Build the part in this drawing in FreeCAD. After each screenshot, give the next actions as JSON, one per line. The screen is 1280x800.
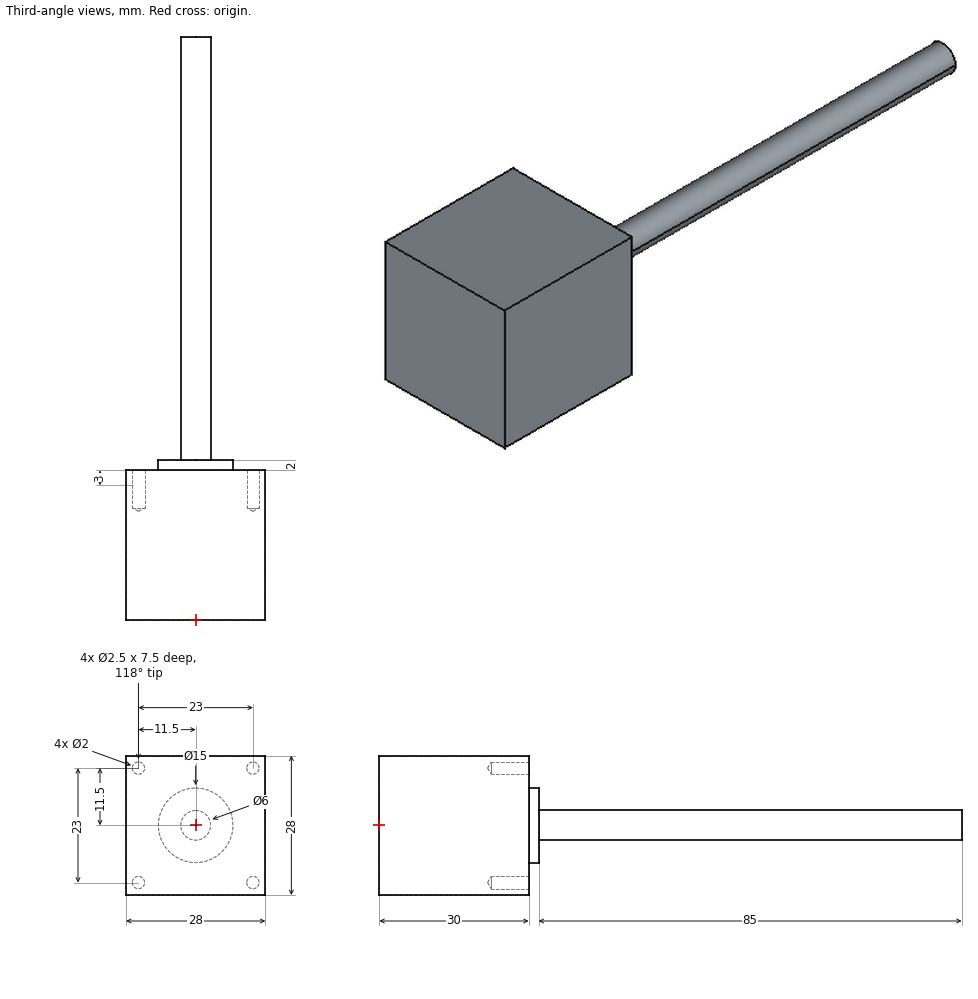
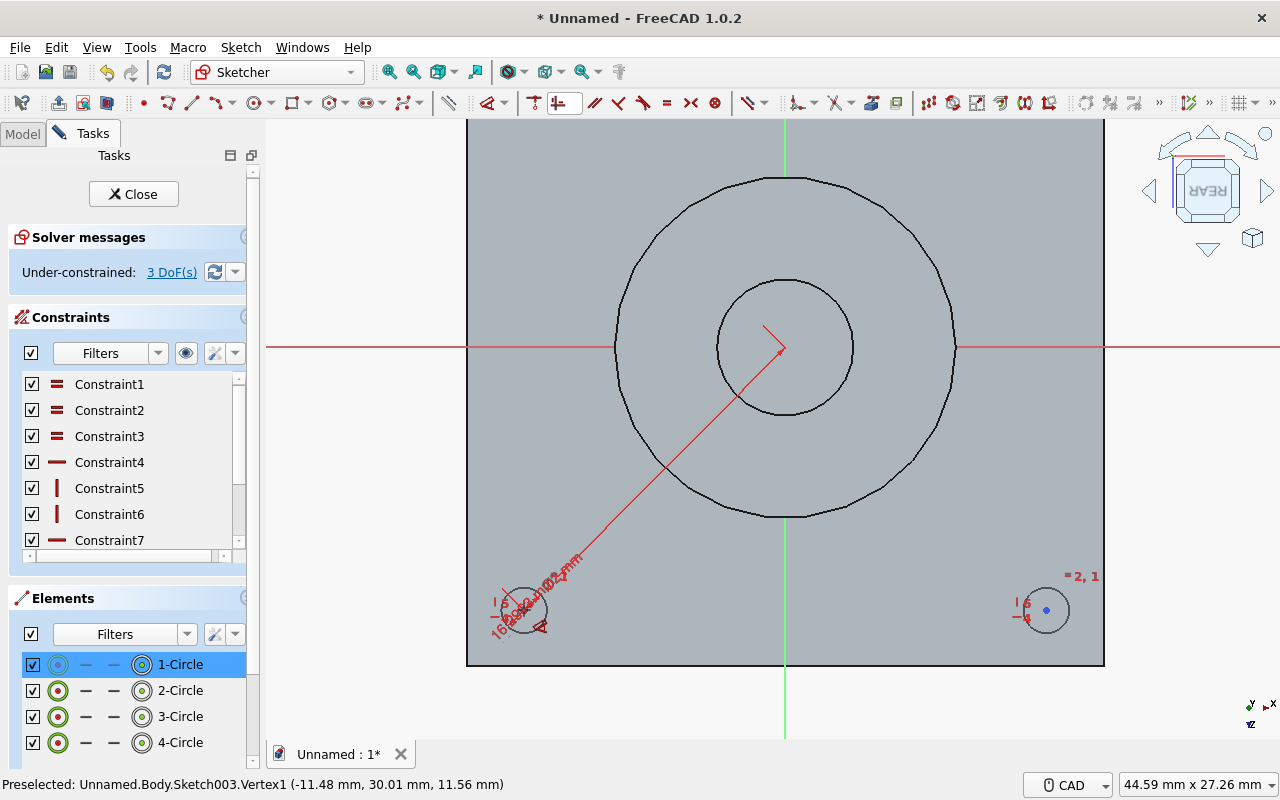
{"action": "left_click", "coordinate": [1046, 610]}
{"action": "left_click", "coordinate": [665, 644]}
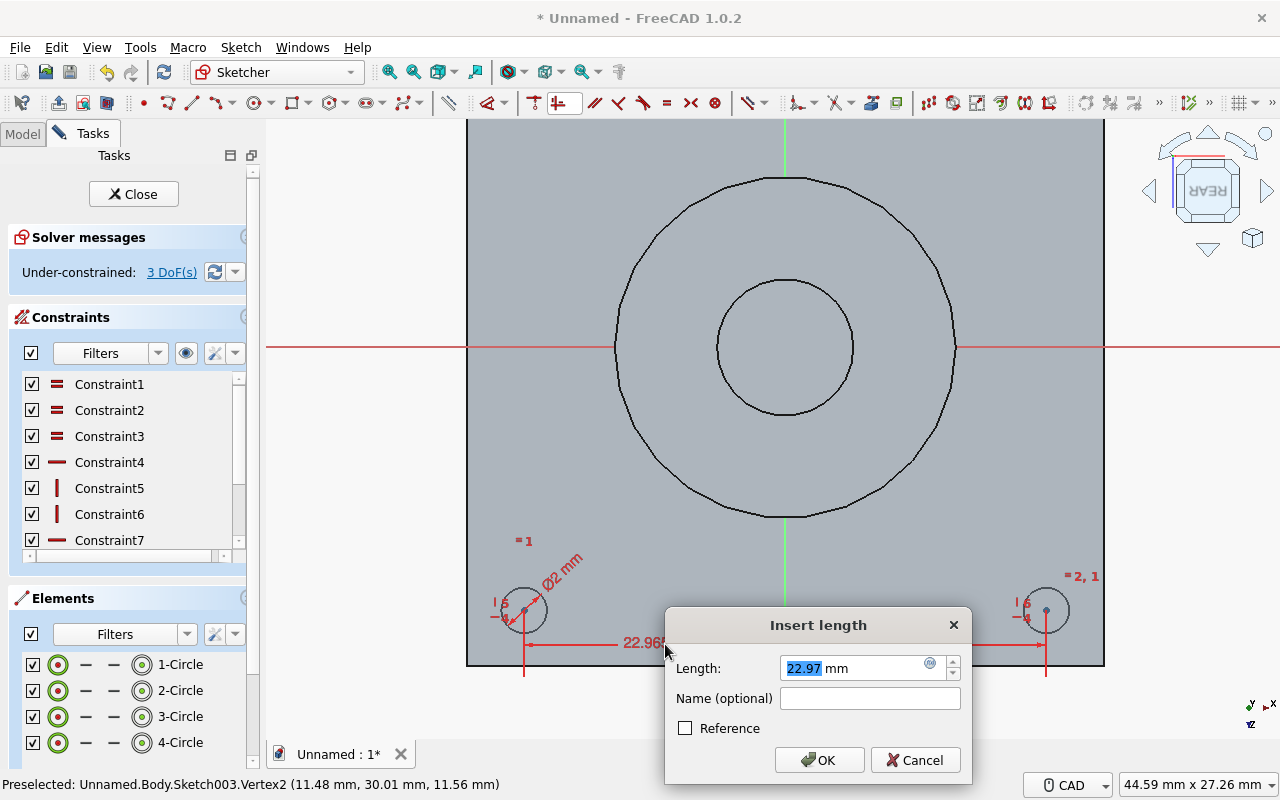
{"action": "type", "text": "23"}
{"action": "key", "text": "Return"}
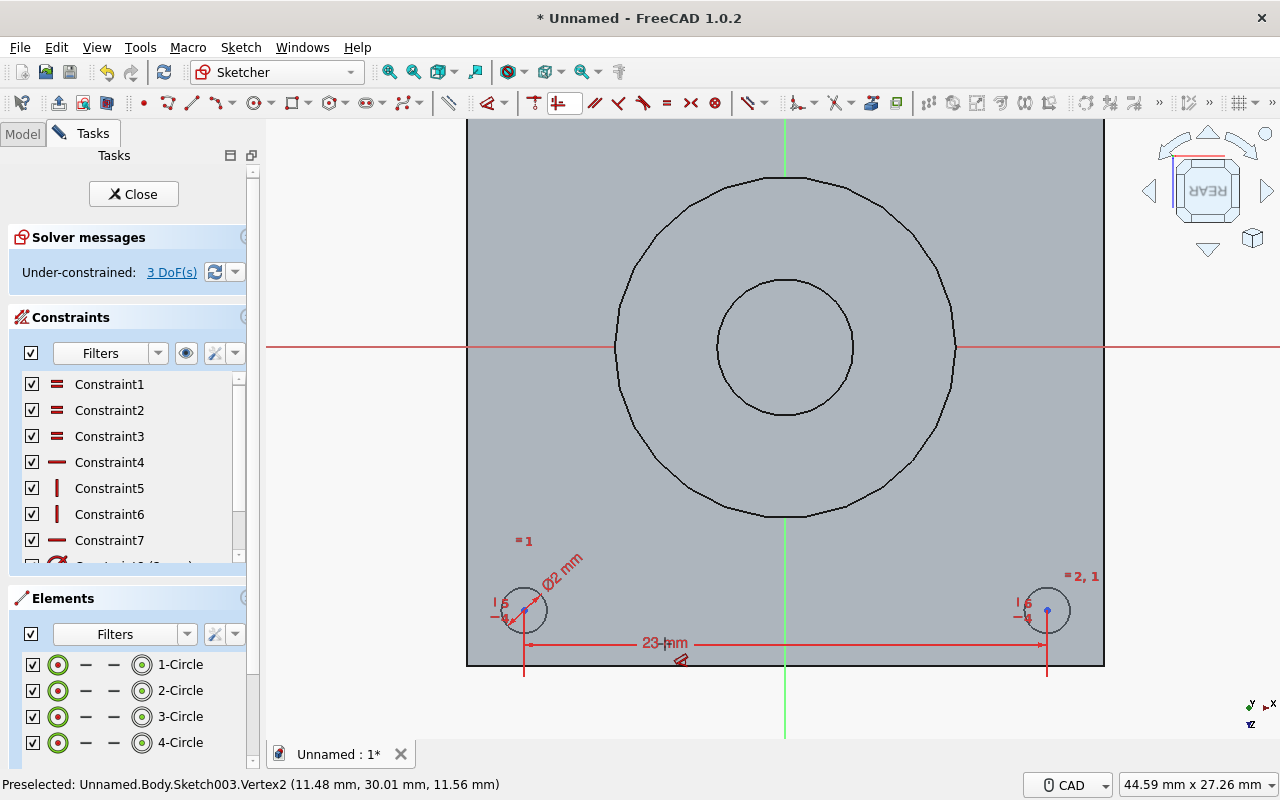
{"action": "left_click", "coordinate": [524, 610]}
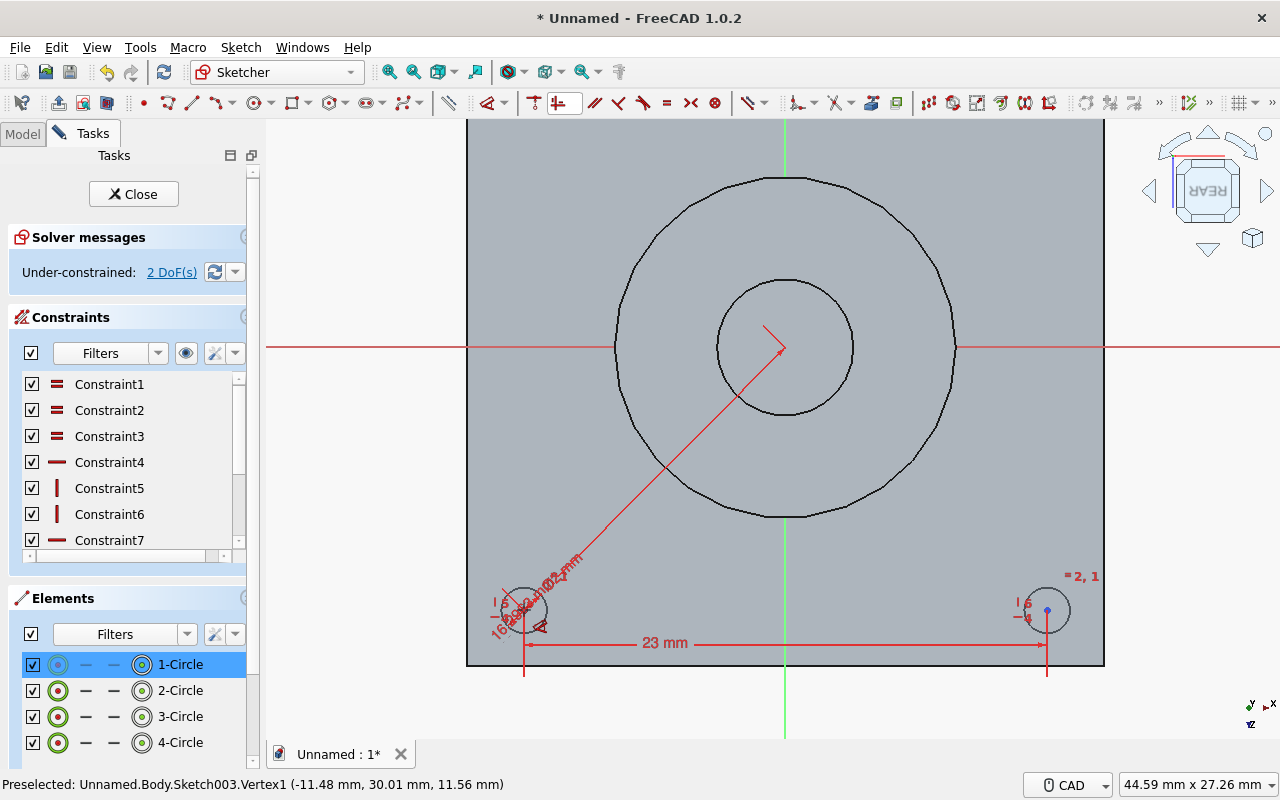
{"action": "scroll", "coordinate": [540, 595], "scroll_direction": "down", "scroll_amount": 2}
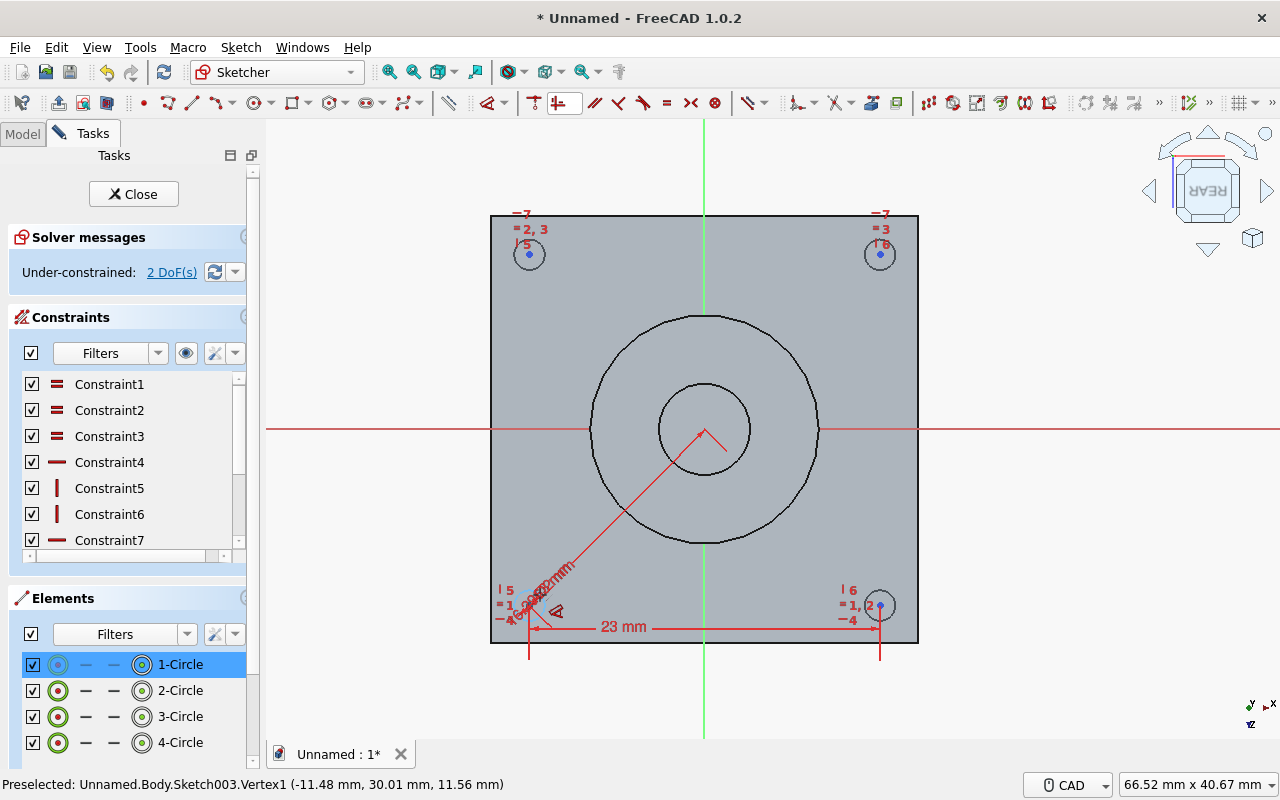
{"action": "left_click", "coordinate": [529, 255]}
{"action": "left_click", "coordinate": [495, 349]}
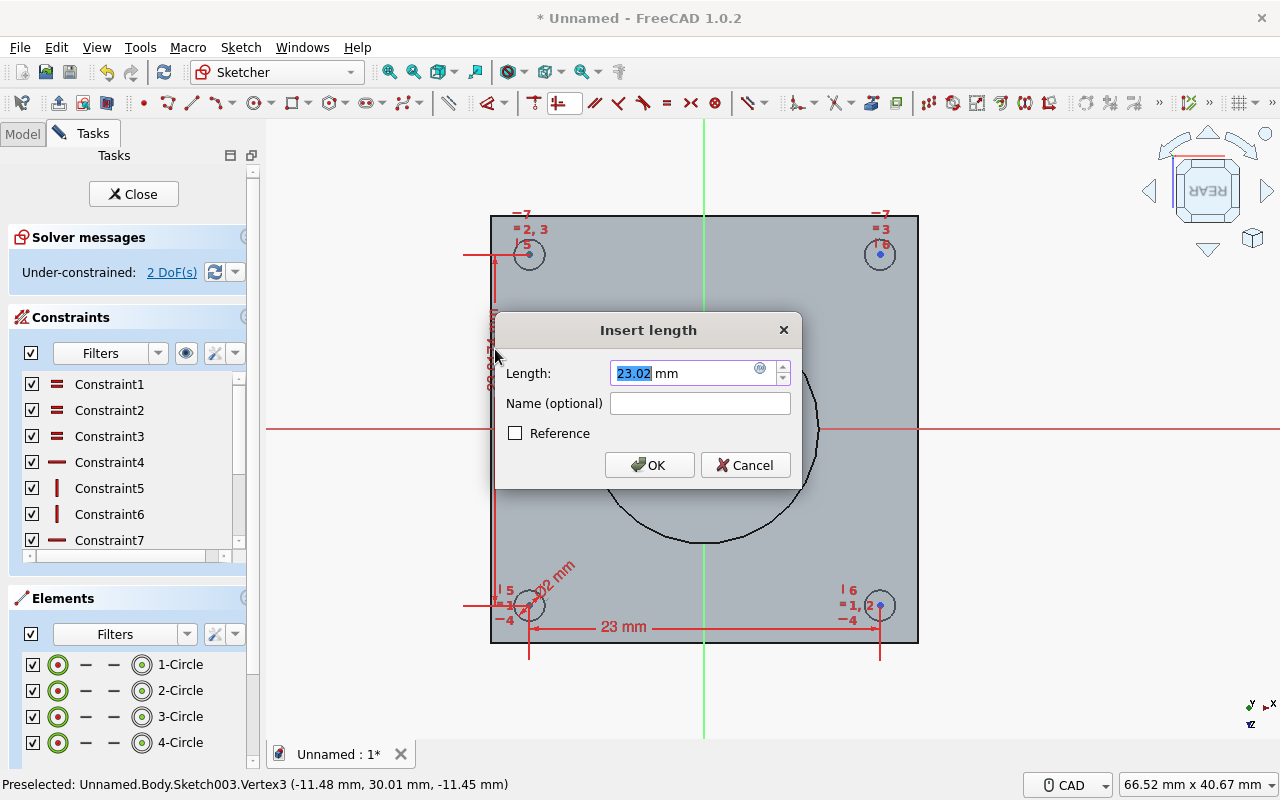
{"action": "type", "text": "23"}
{"action": "key", "text": "Return"}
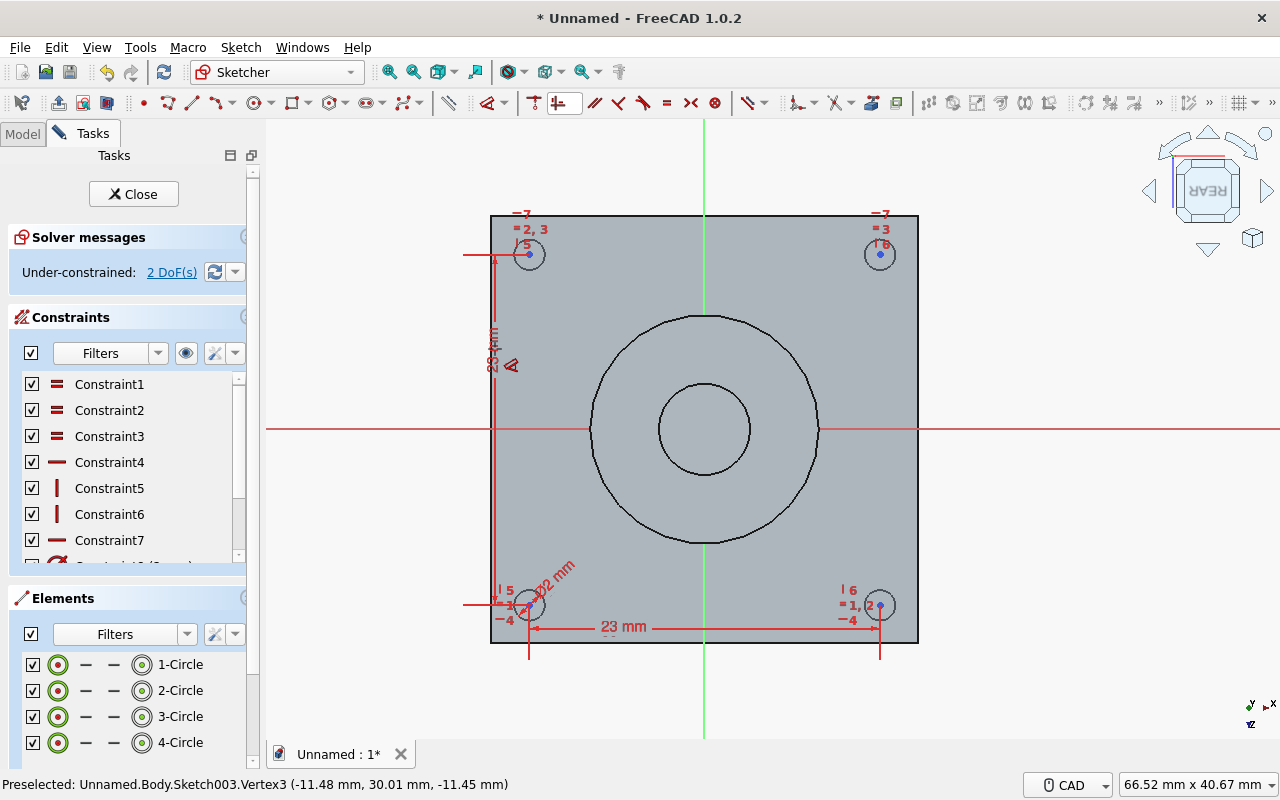
{"action": "left_click", "coordinate": [529, 605]}
{"action": "left_click", "coordinate": [617, 395]}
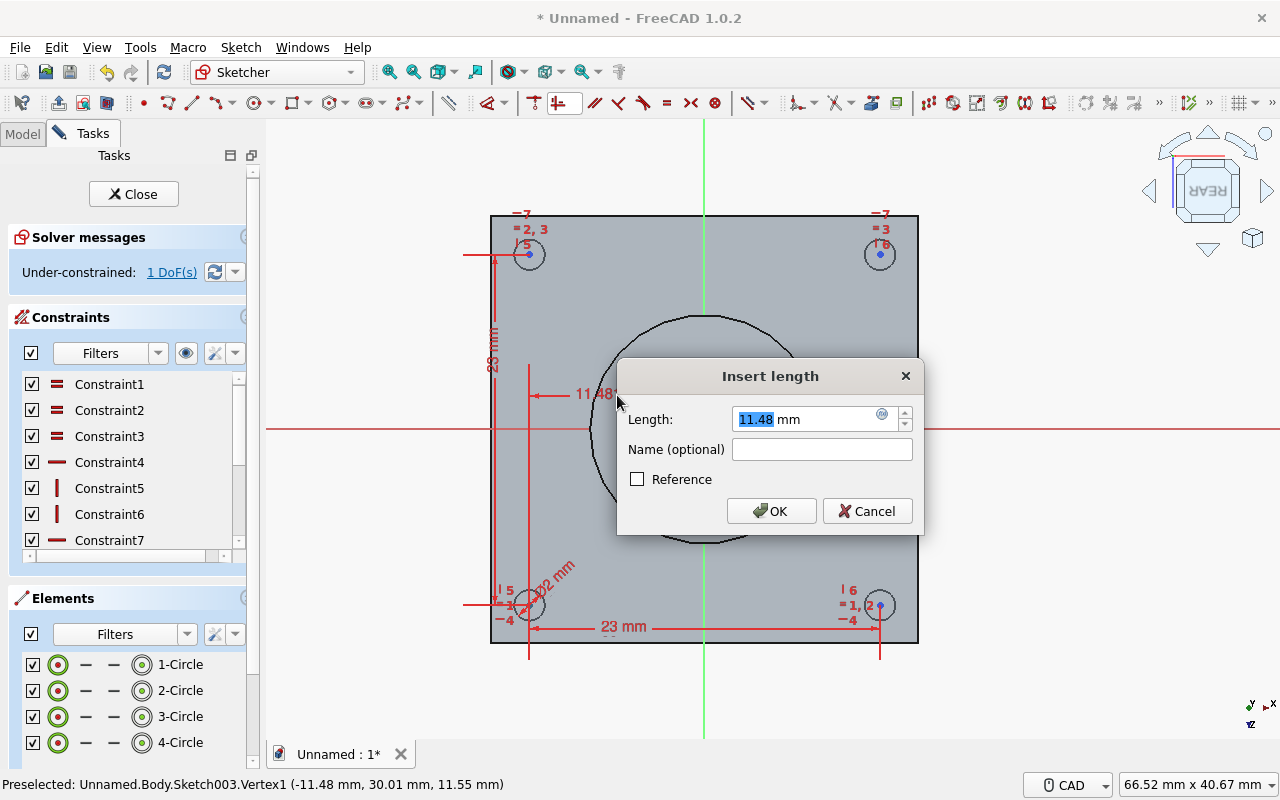
{"action": "type", "text": "11.5"}
{"action": "key", "text": "Return"}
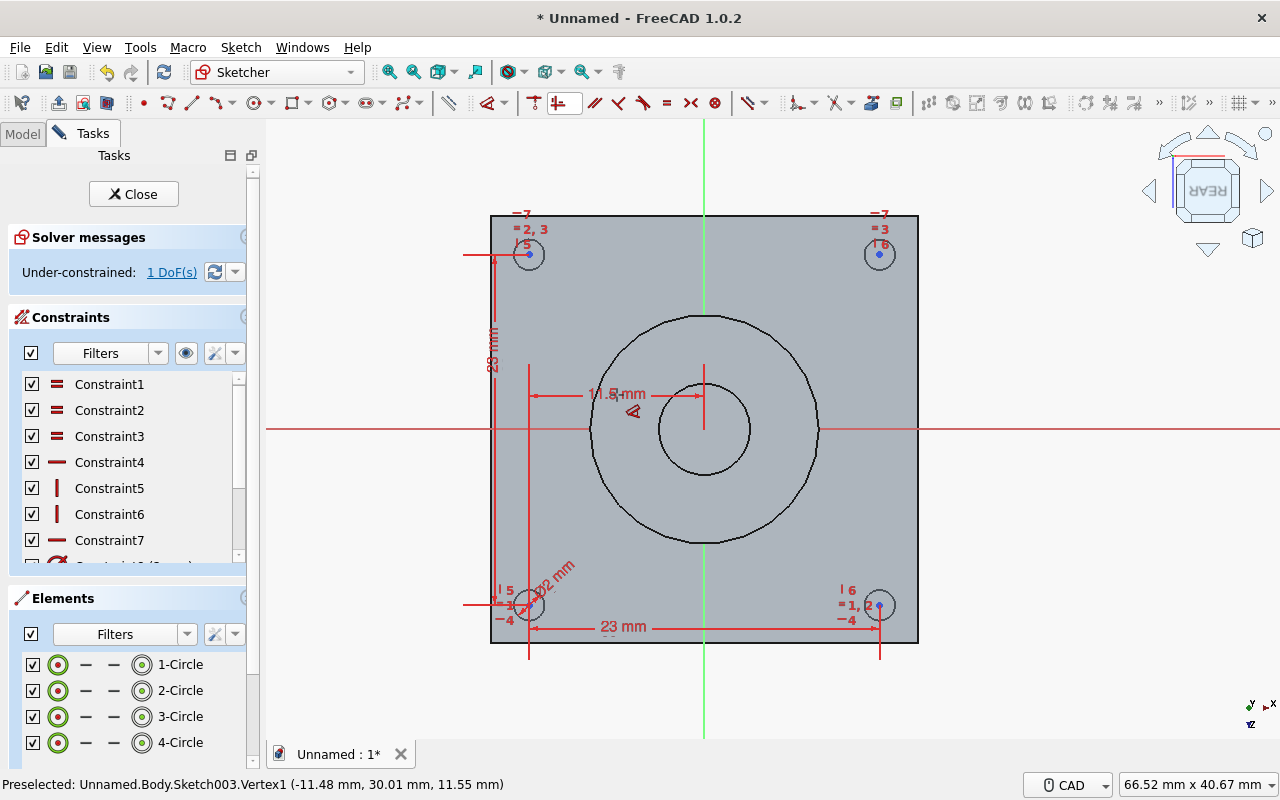
{"action": "left_click", "coordinate": [529, 605]}
{"action": "left_click", "coordinate": [495, 517]}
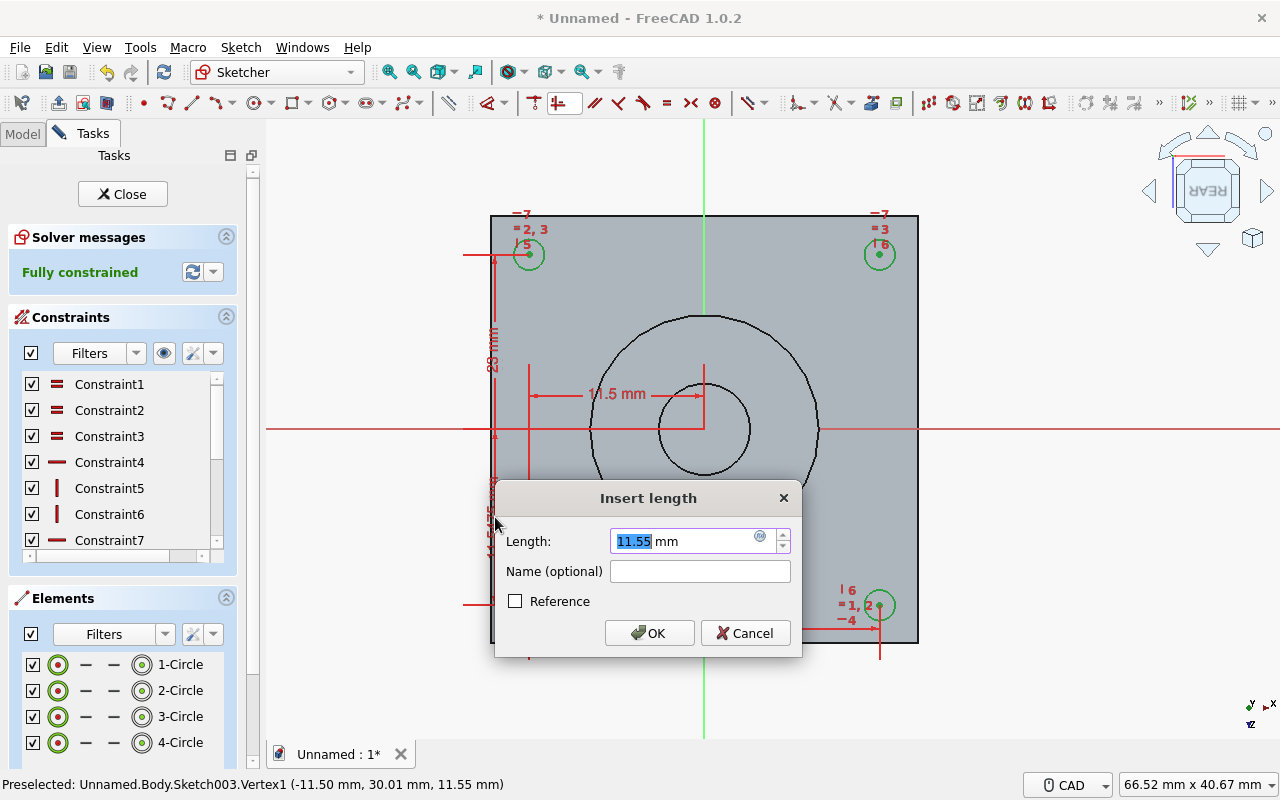
{"action": "type", "text": "11.5"}
{"action": "key", "text": "Return"}
{"action": "key", "text": "Escape"}